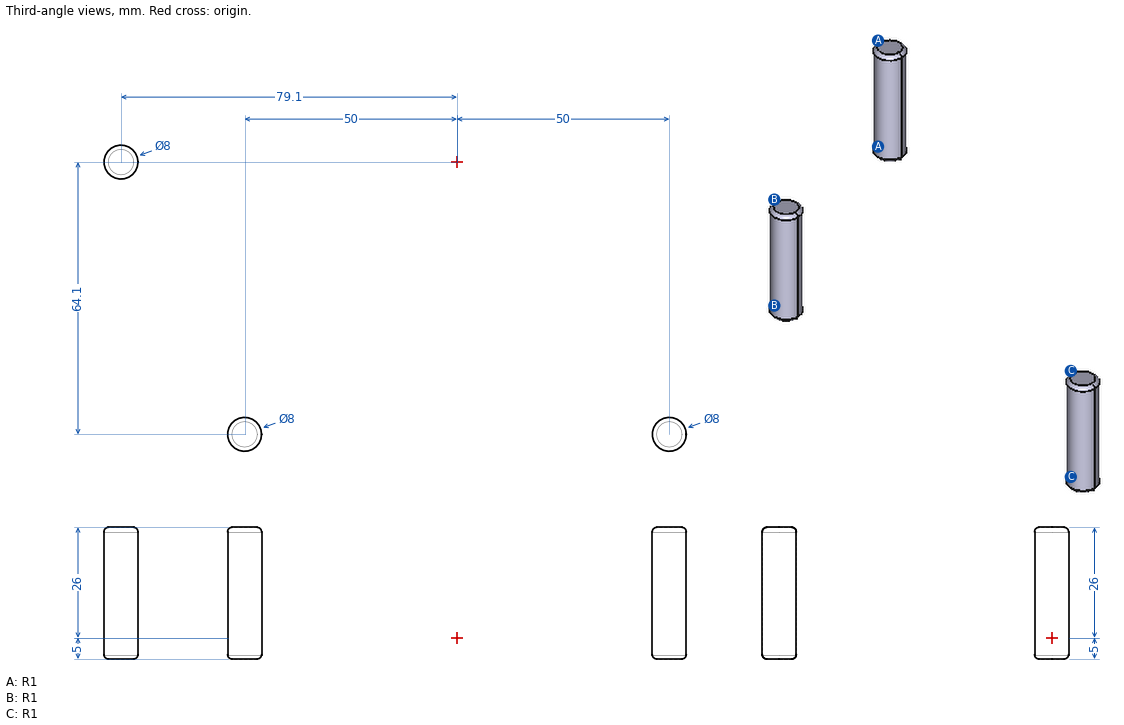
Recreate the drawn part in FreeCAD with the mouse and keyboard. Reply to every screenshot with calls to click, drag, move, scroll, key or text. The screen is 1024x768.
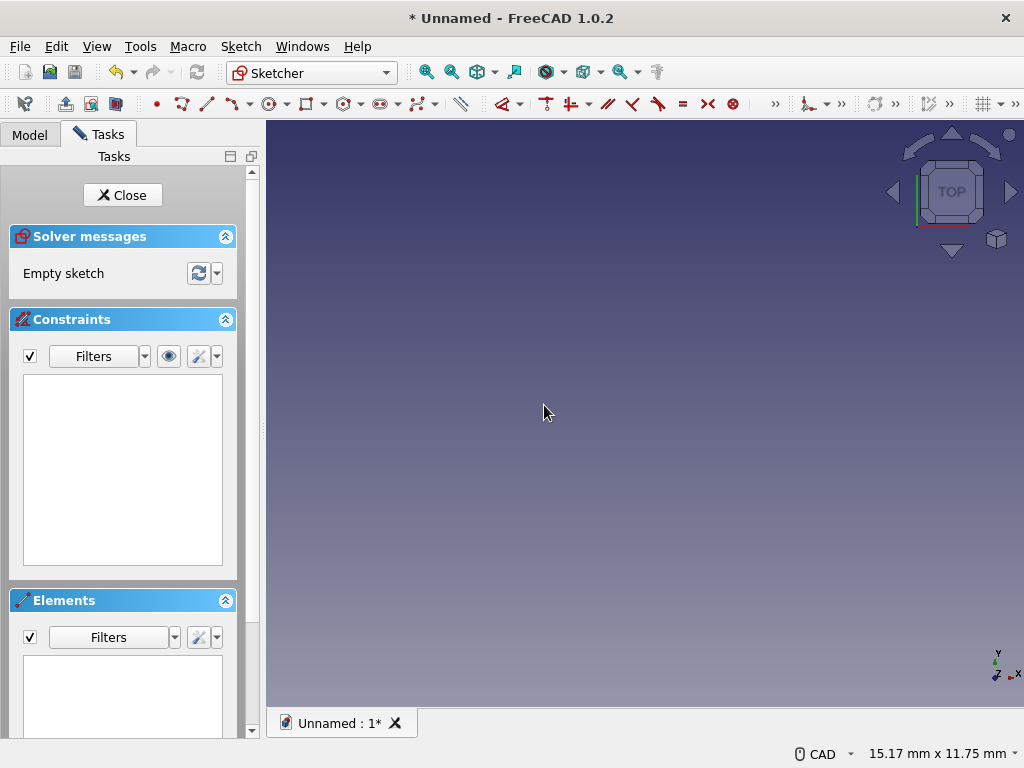
click(268, 104)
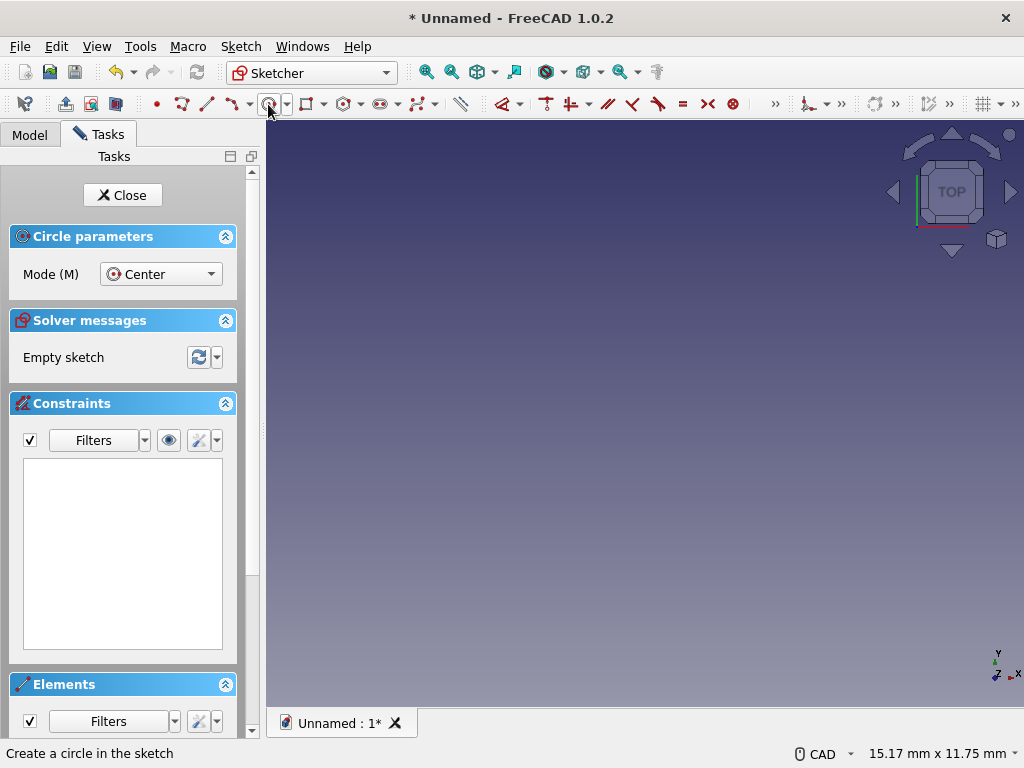
click(576, 413)
click(718, 272)
key(Escape)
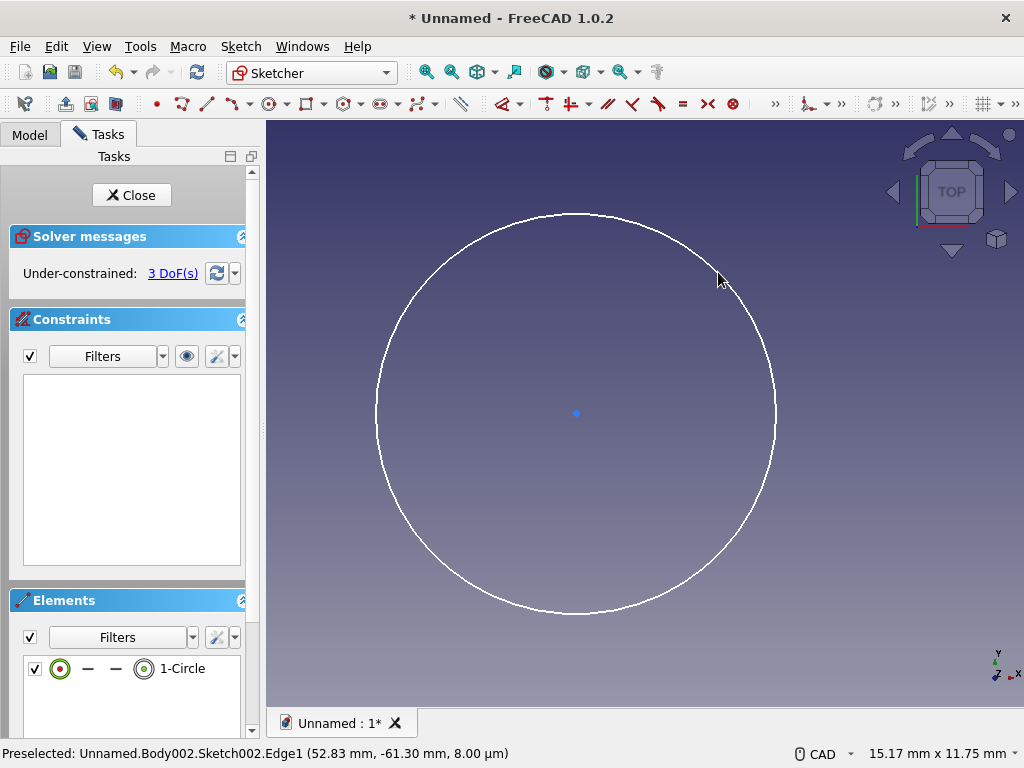
click(502, 104)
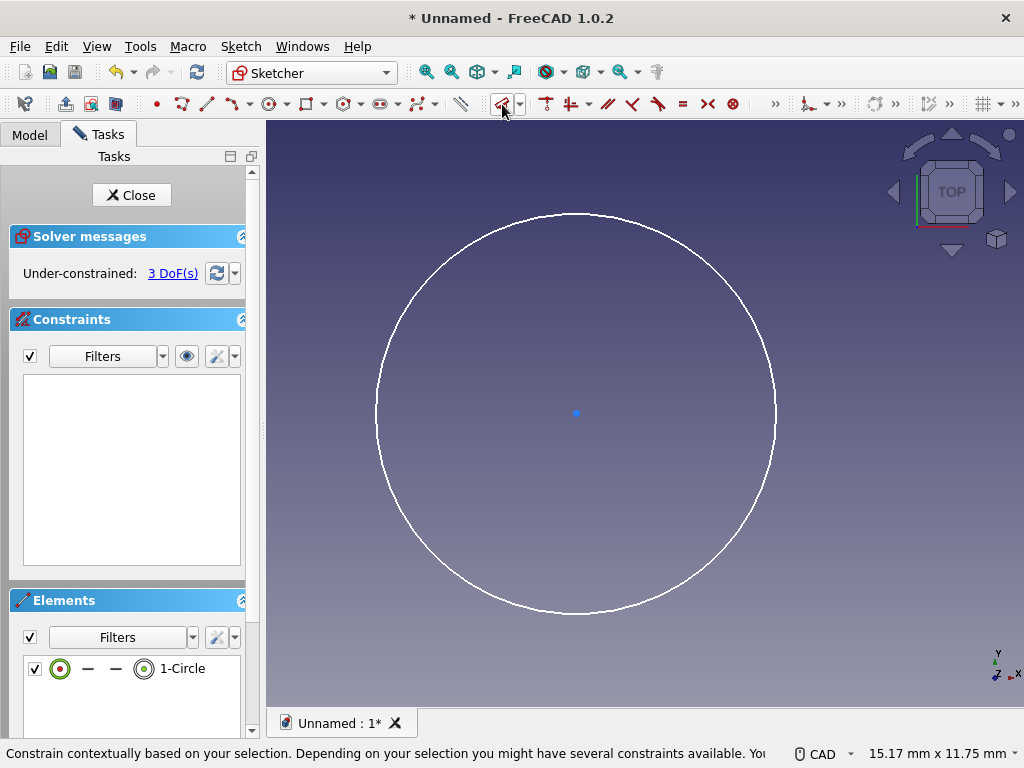
click(717, 272)
click(740, 249)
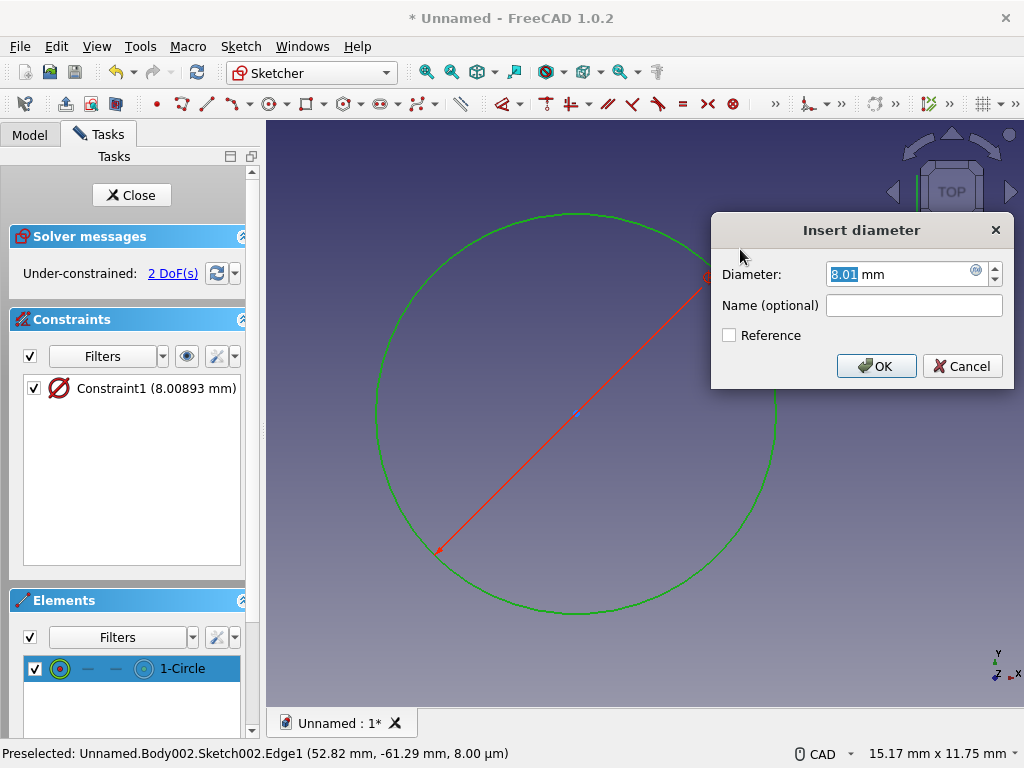
text(8)
key(Return)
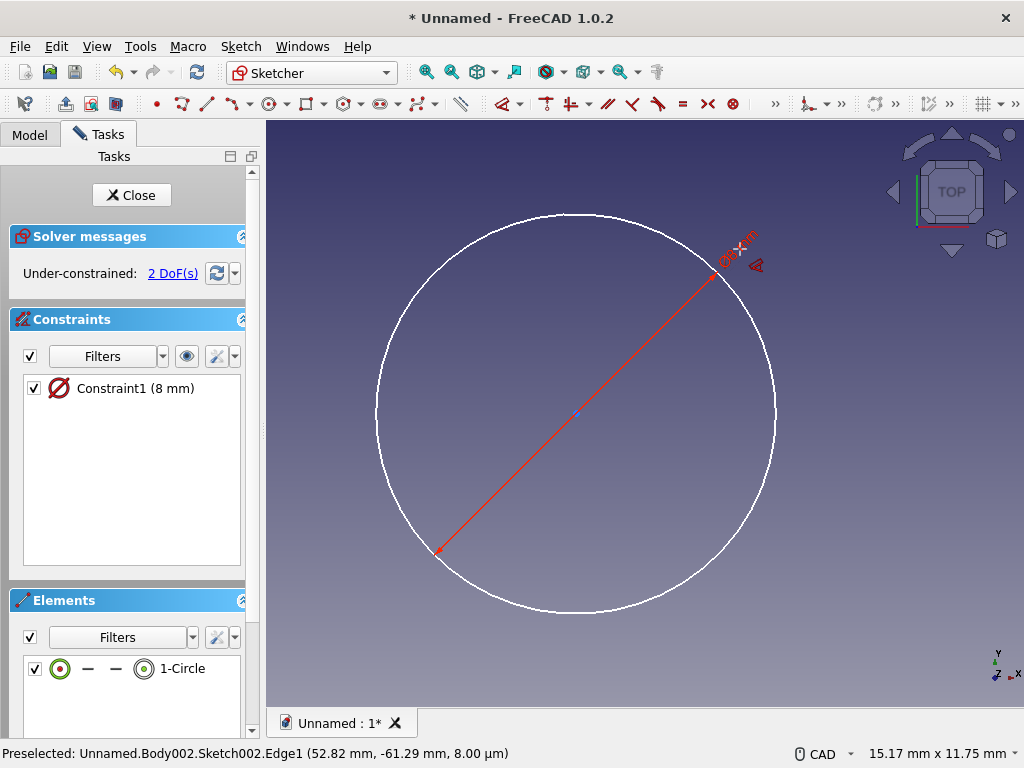
click(576, 414)
click(435, 448)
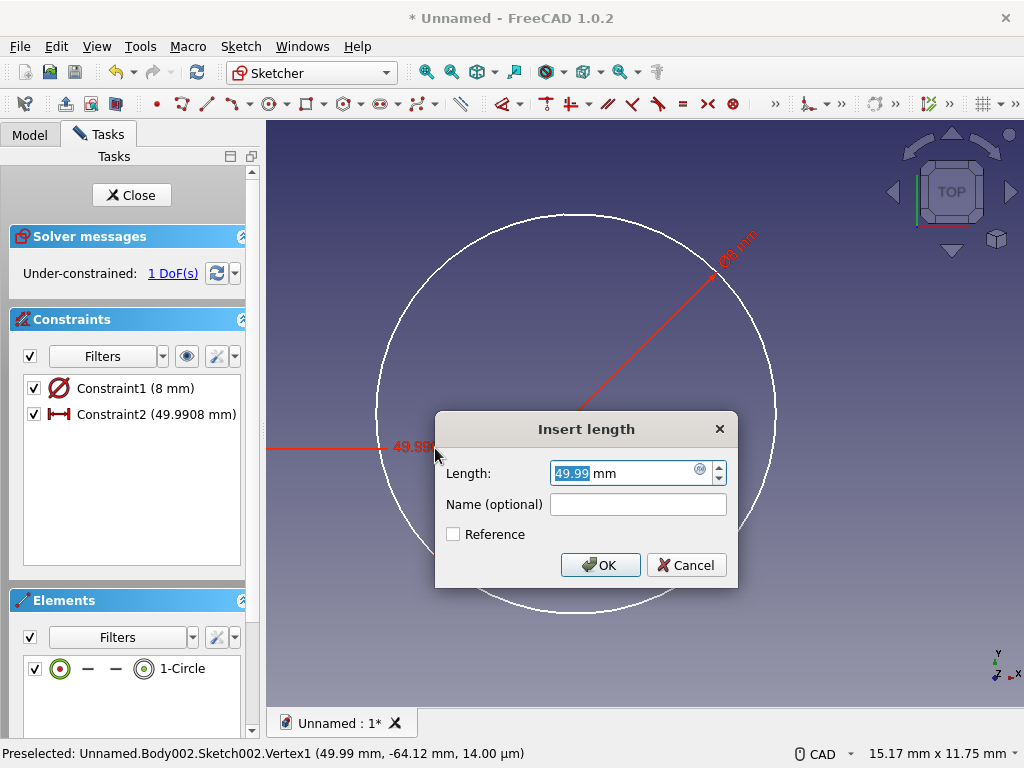
text(50)
key(Return)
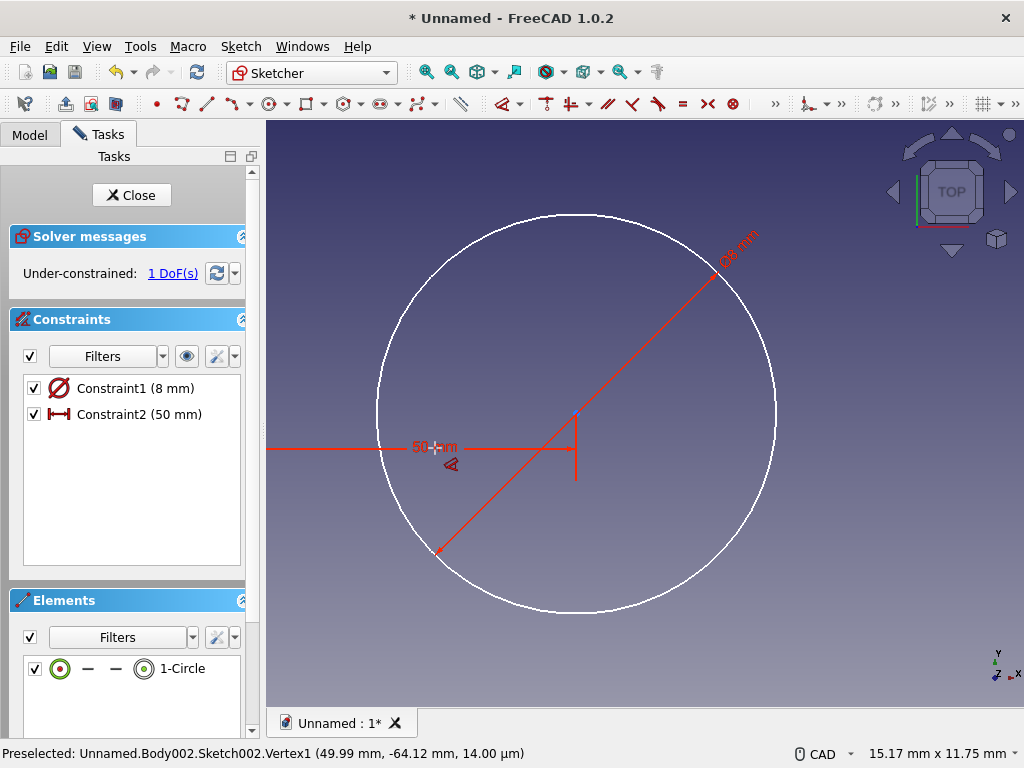
click(576, 414)
click(610, 281)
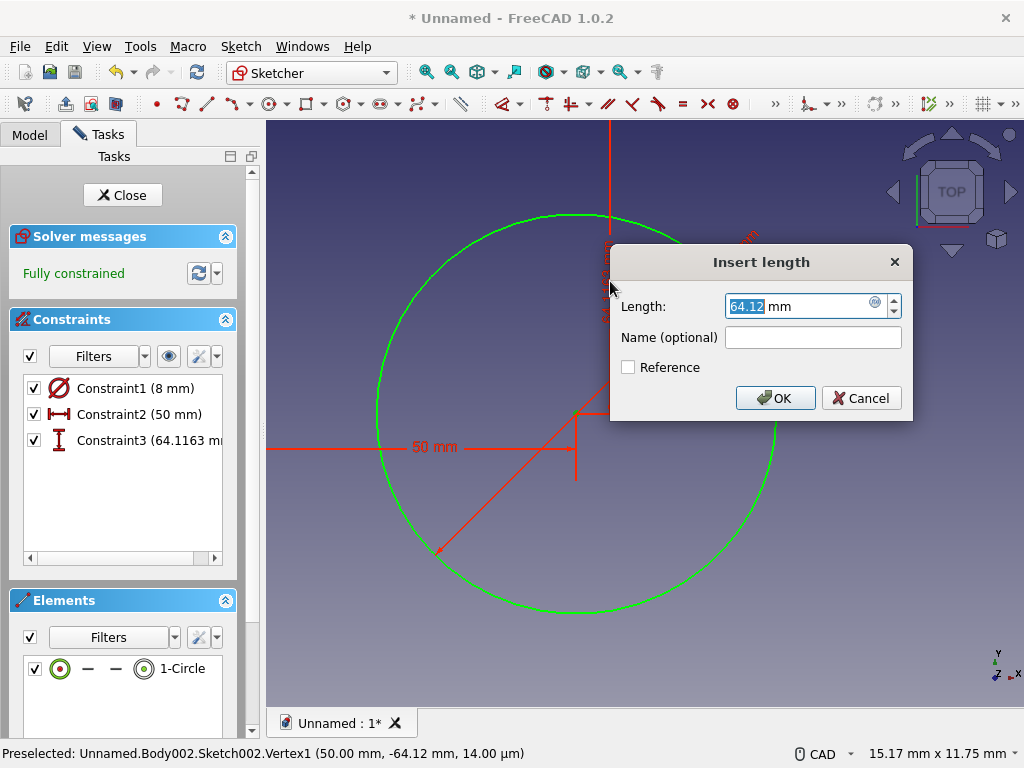
text(64.1)
key(Return)
key(Escape)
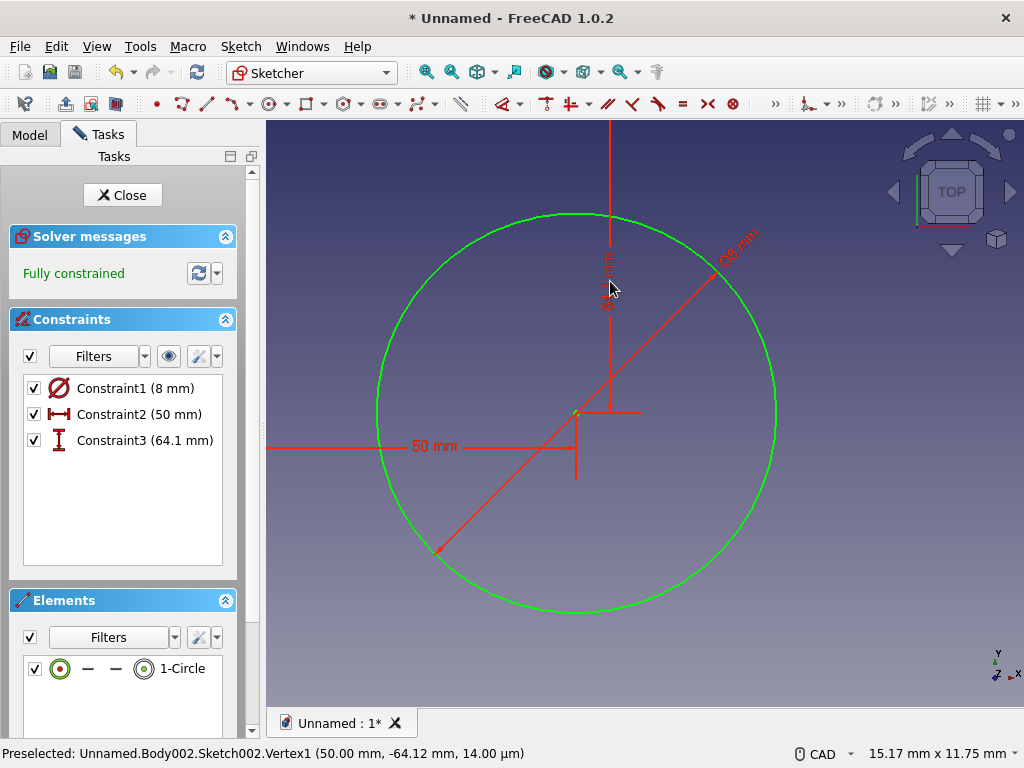
click(123, 195)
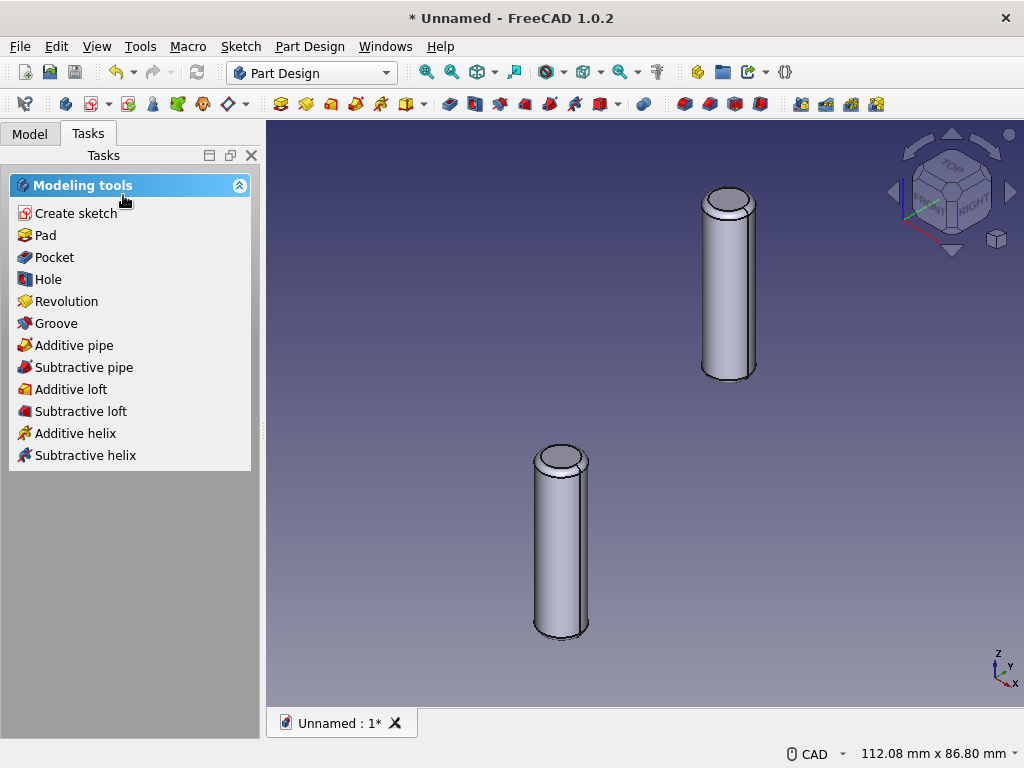
click(281, 104)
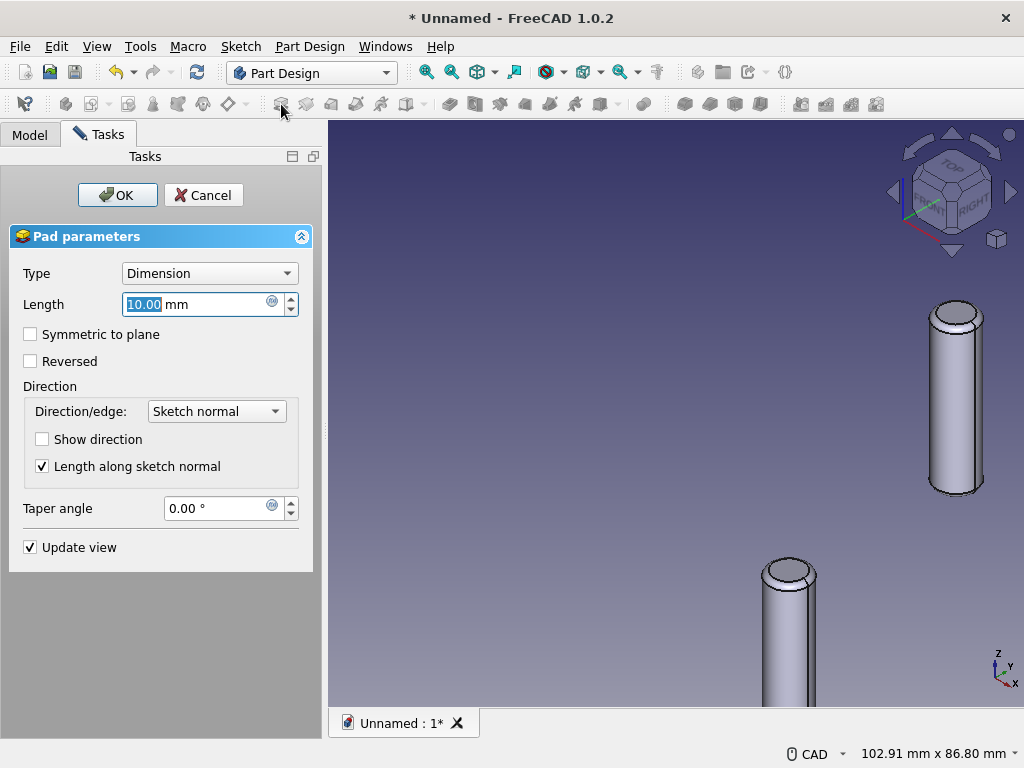
click(210, 274)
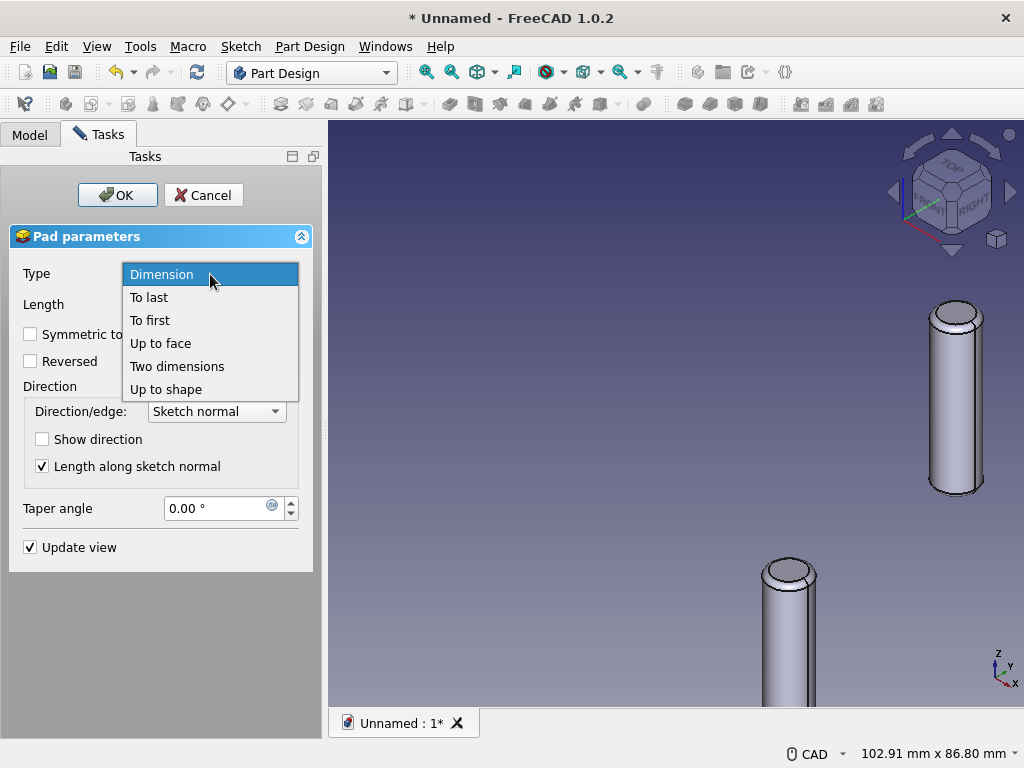
click(208, 366)